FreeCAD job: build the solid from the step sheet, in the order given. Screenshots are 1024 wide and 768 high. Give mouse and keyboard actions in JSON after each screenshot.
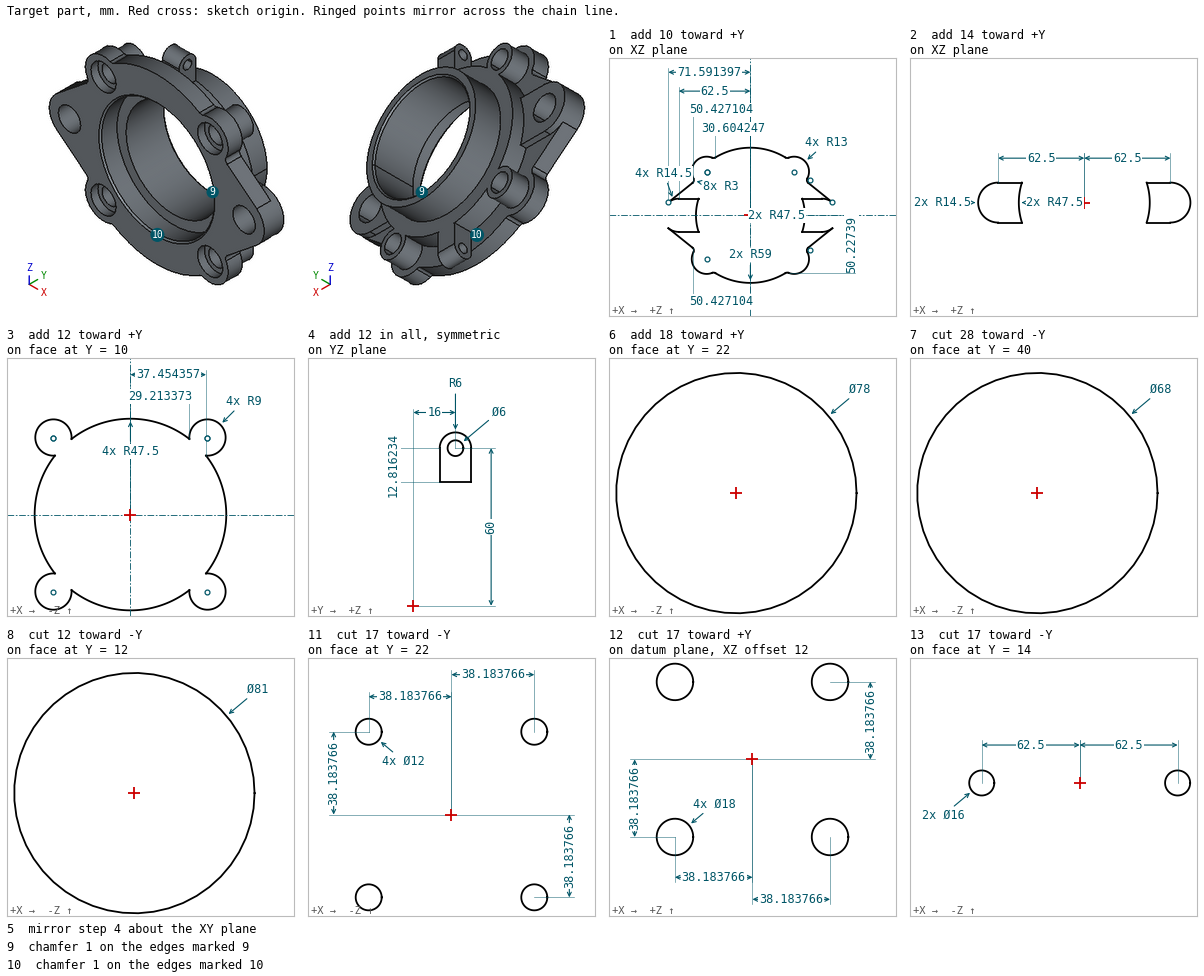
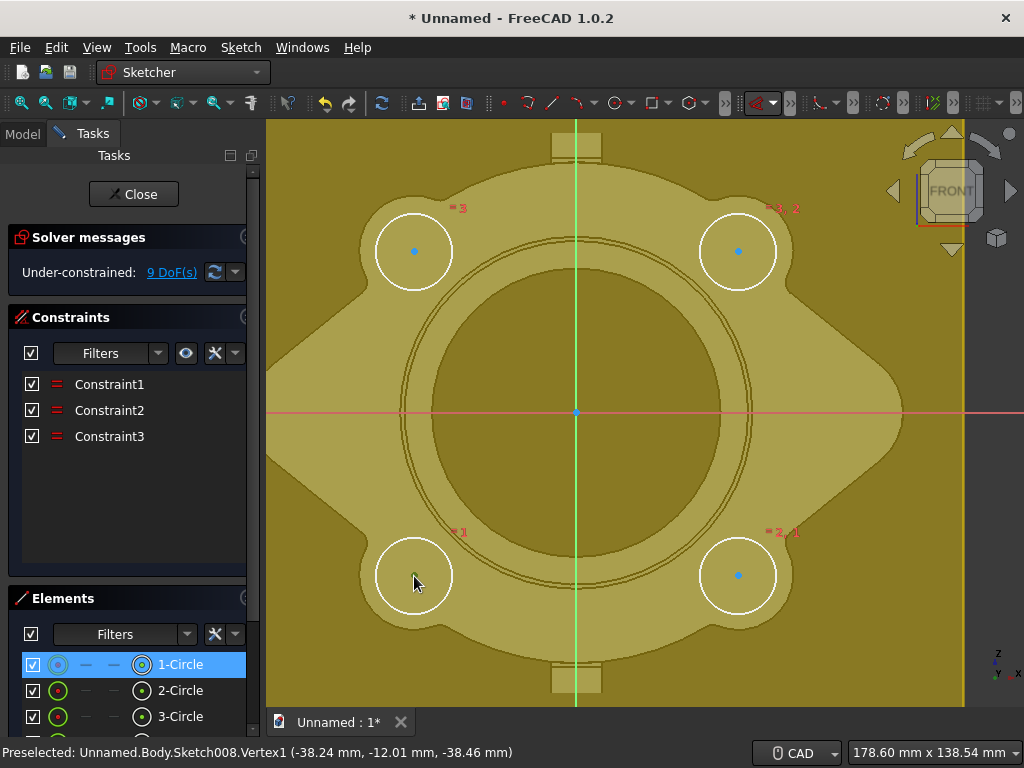
{"action": "left_click", "coordinate": [738, 576]}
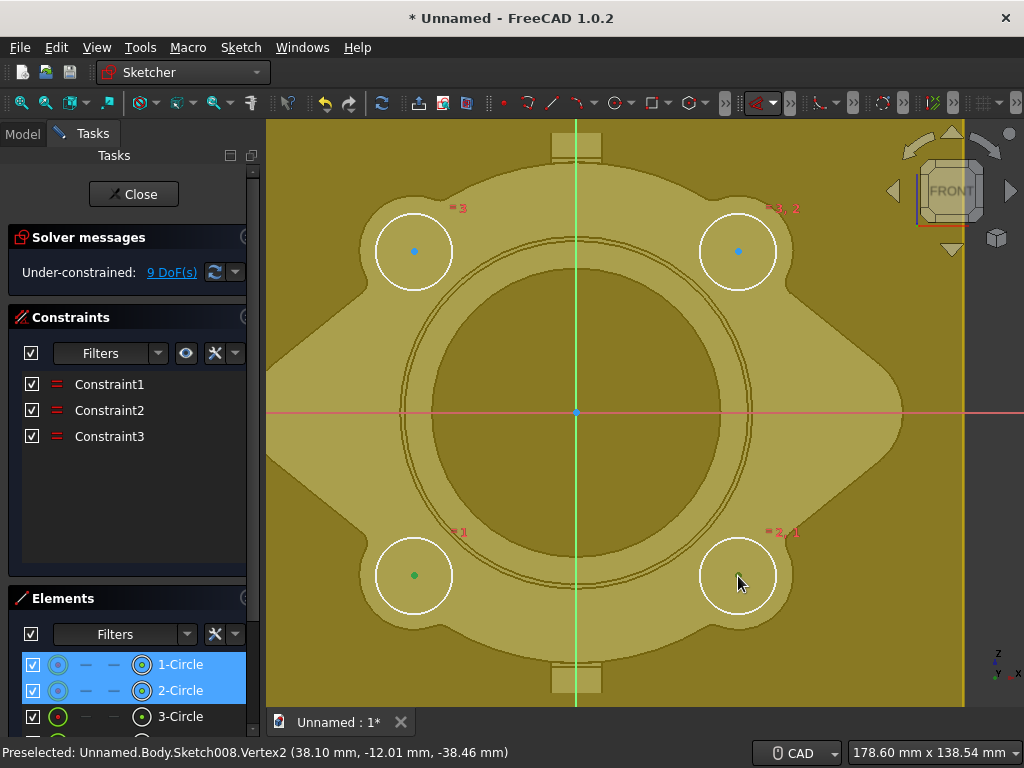
{"action": "key", "text": "h"}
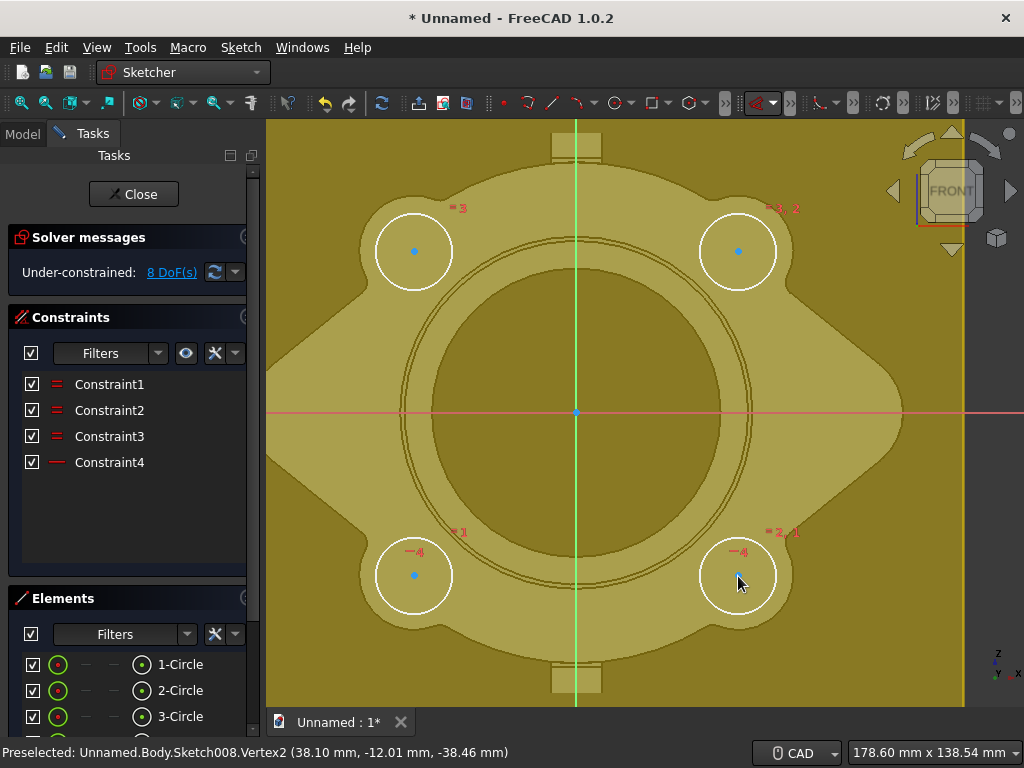
{"action": "left_click", "coordinate": [738, 576]}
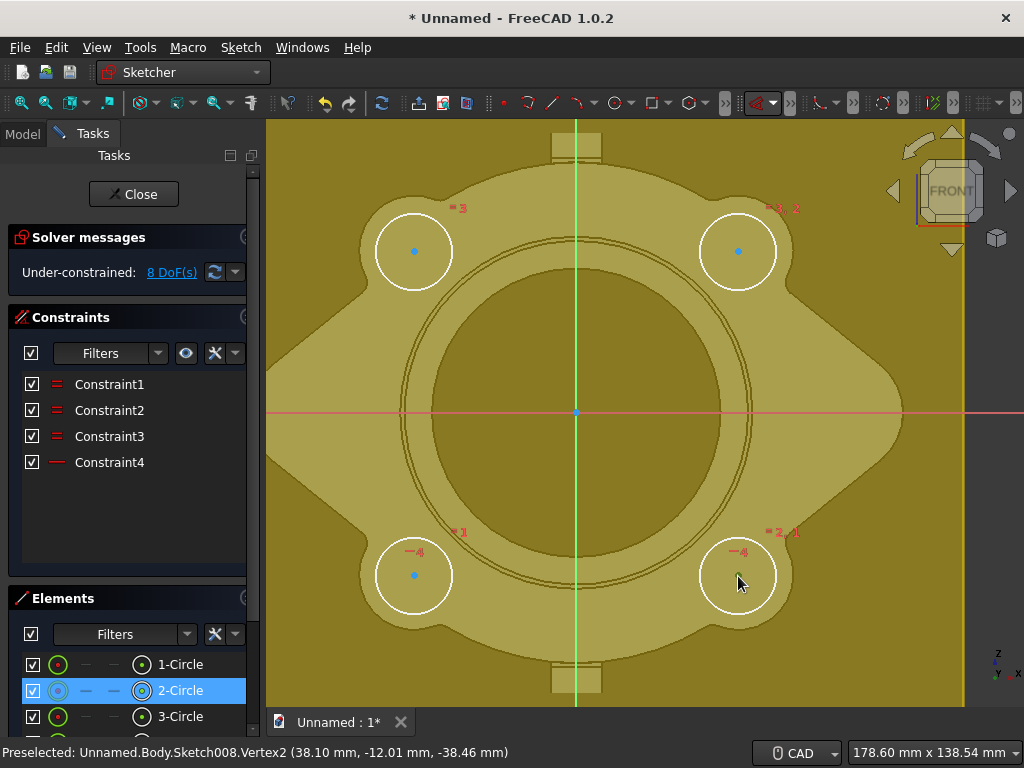
{"action": "left_click", "coordinate": [738, 252]}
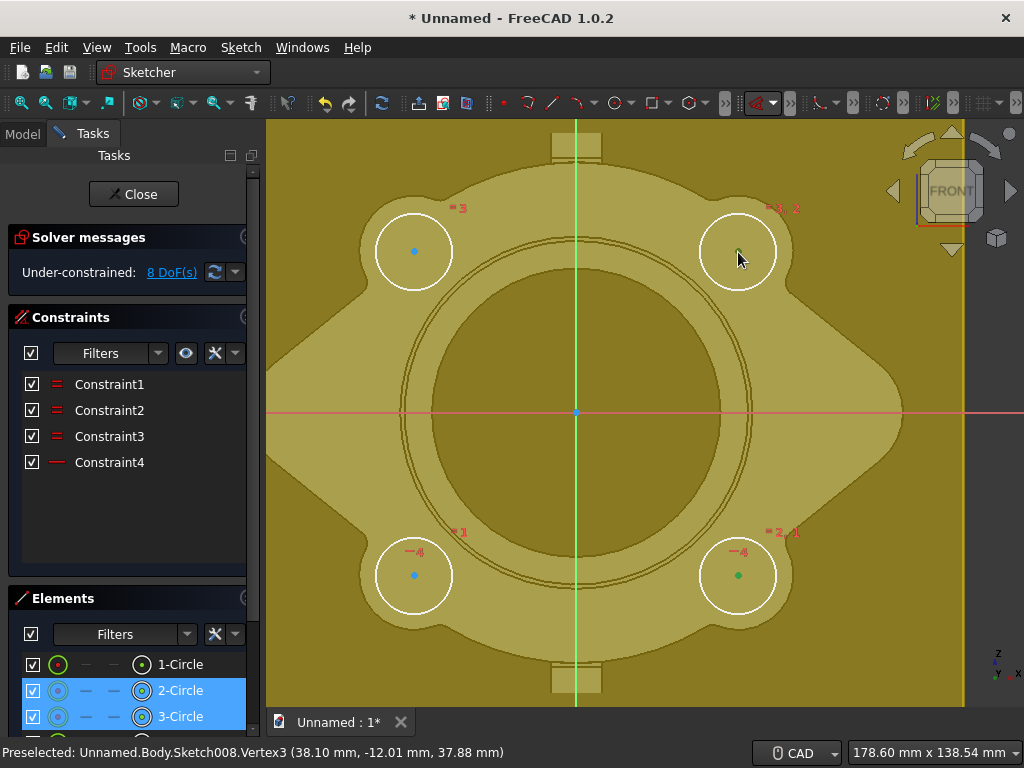
{"action": "key", "text": "v"}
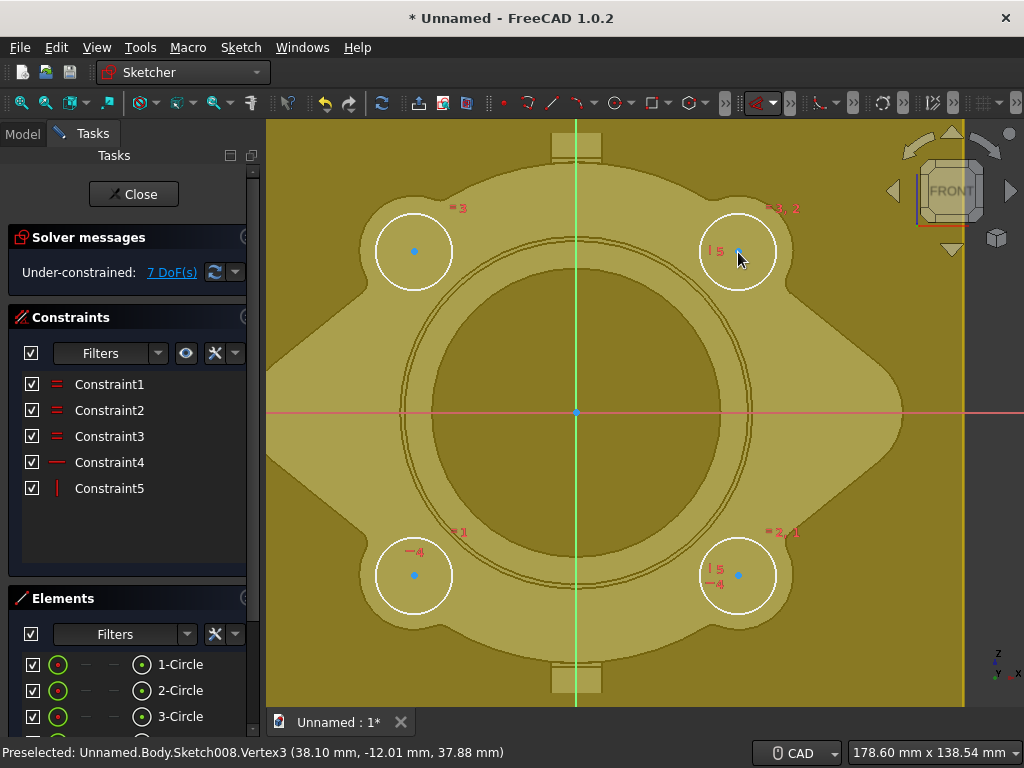
{"action": "left_click", "coordinate": [414, 576]}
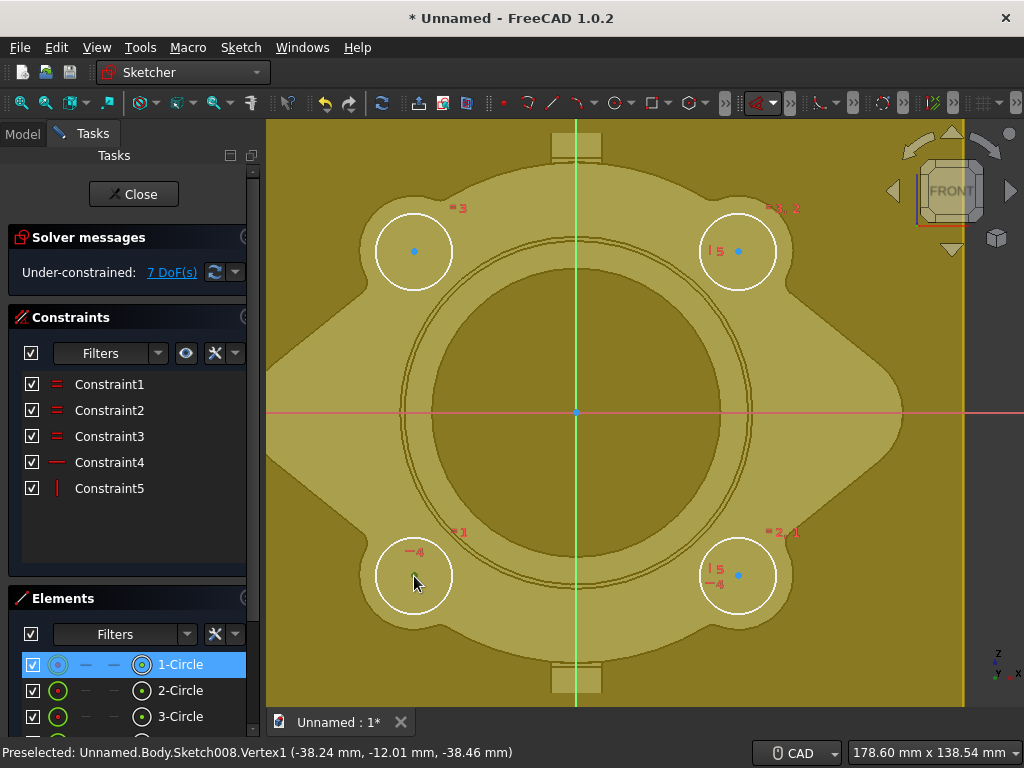
{"action": "left_click", "coordinate": [414, 252]}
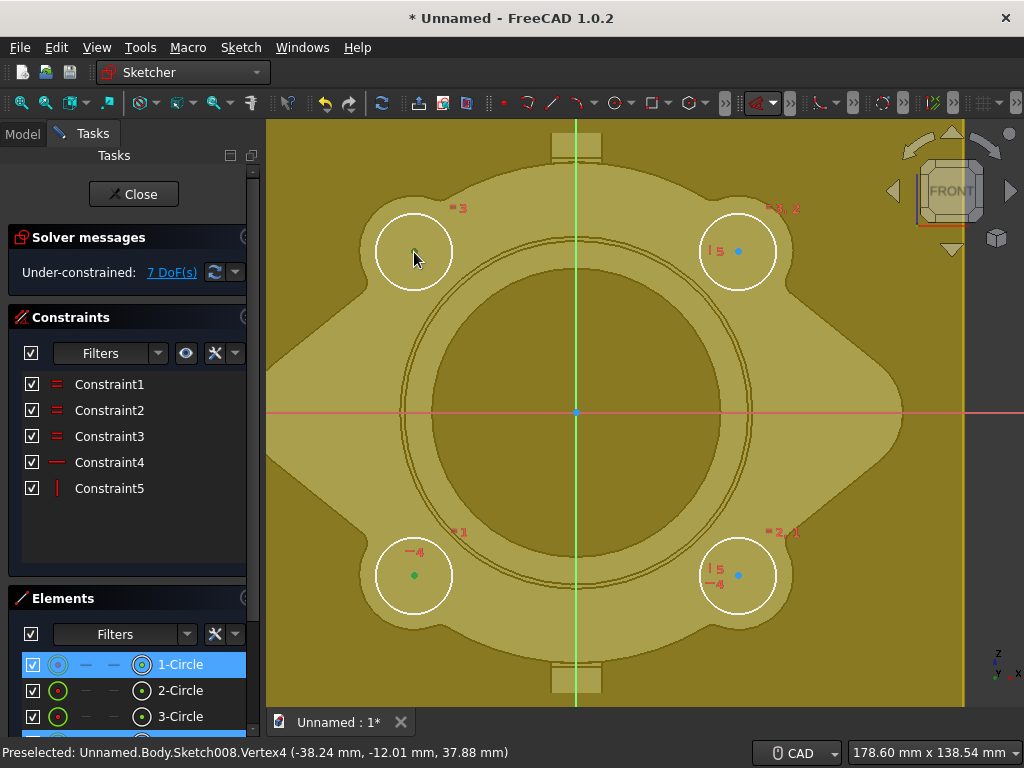
{"action": "key", "text": "v"}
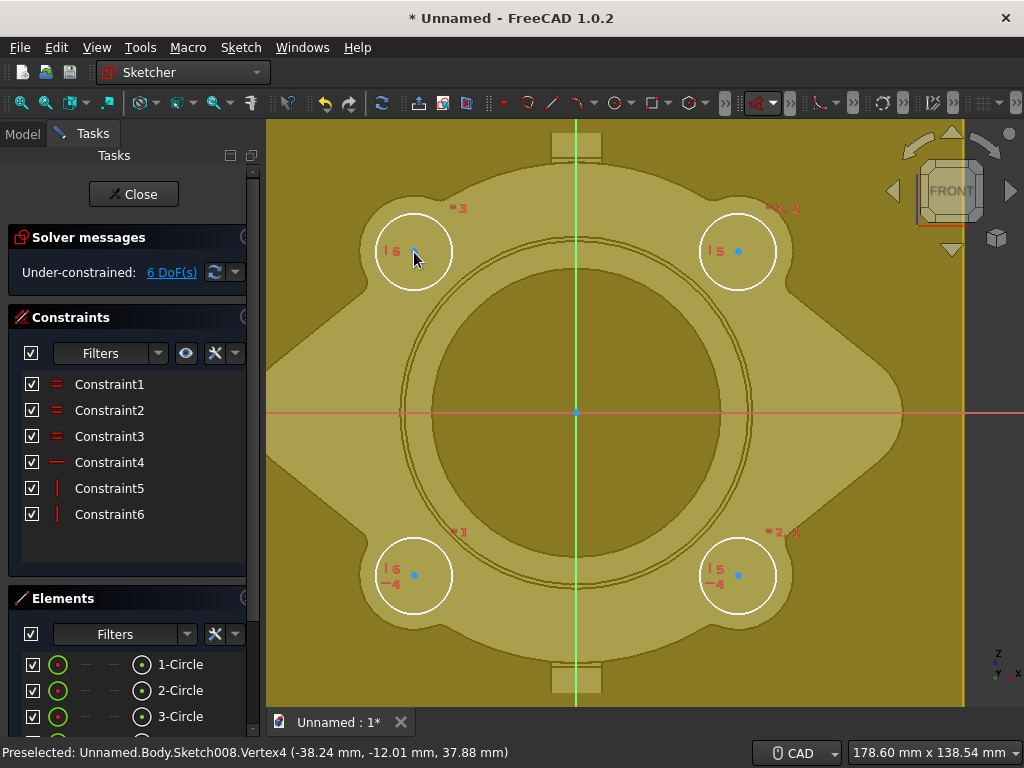
{"action": "left_click", "coordinate": [738, 252]}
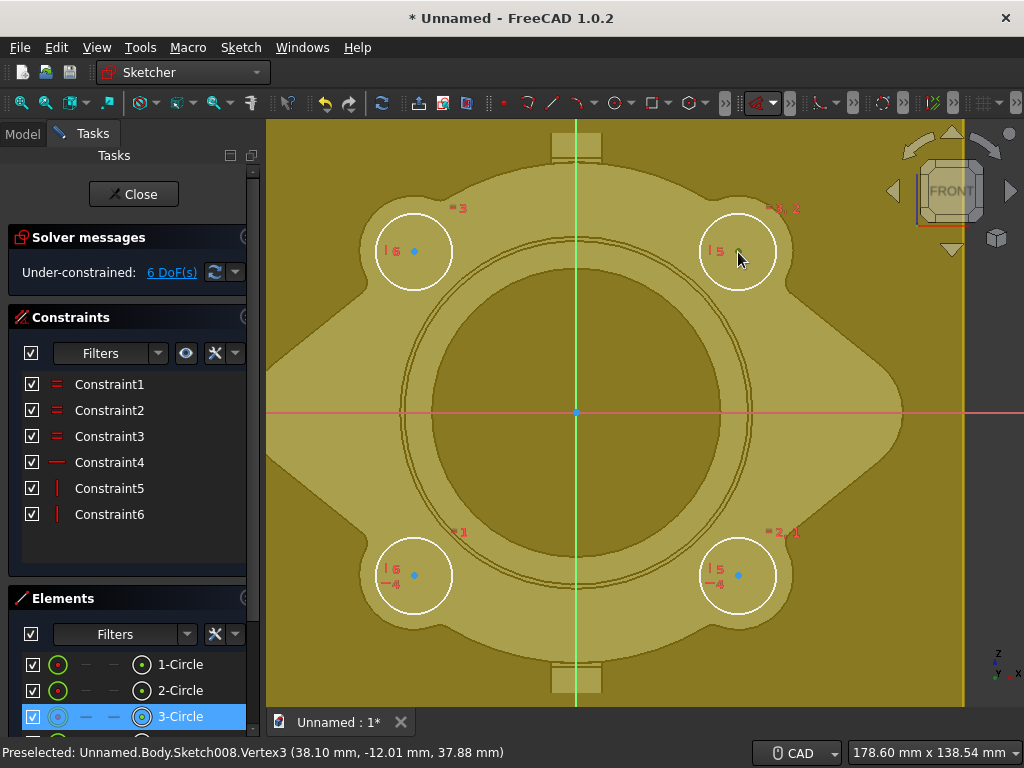
{"action": "left_click", "coordinate": [414, 252]}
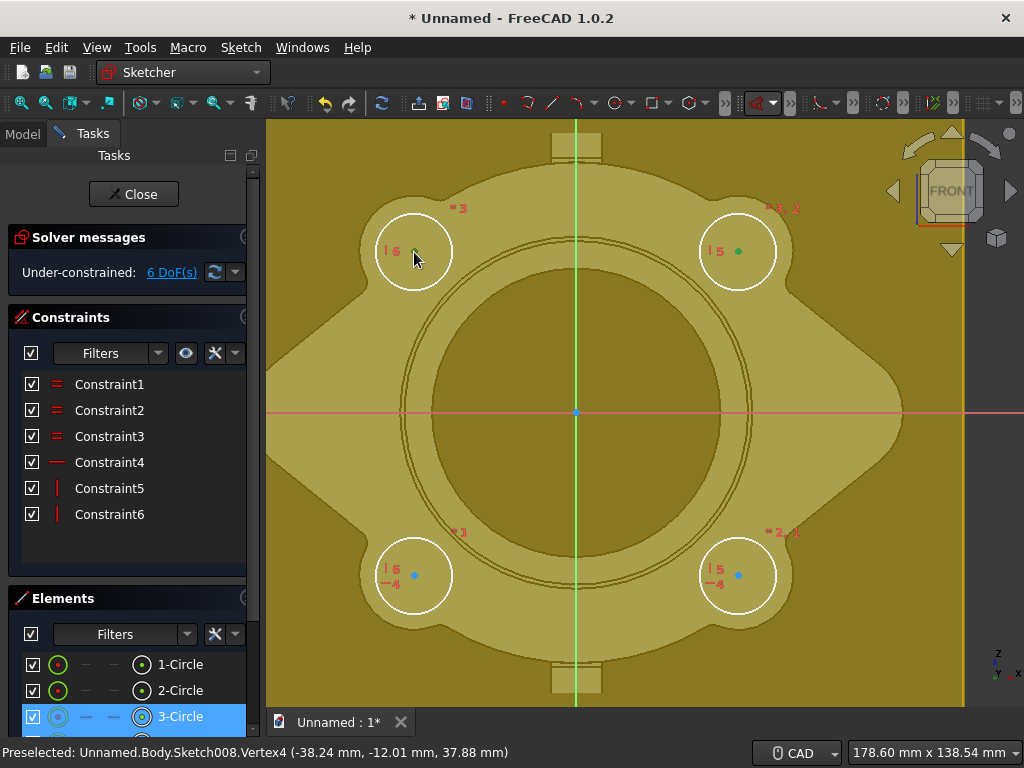
{"action": "key", "text": "h"}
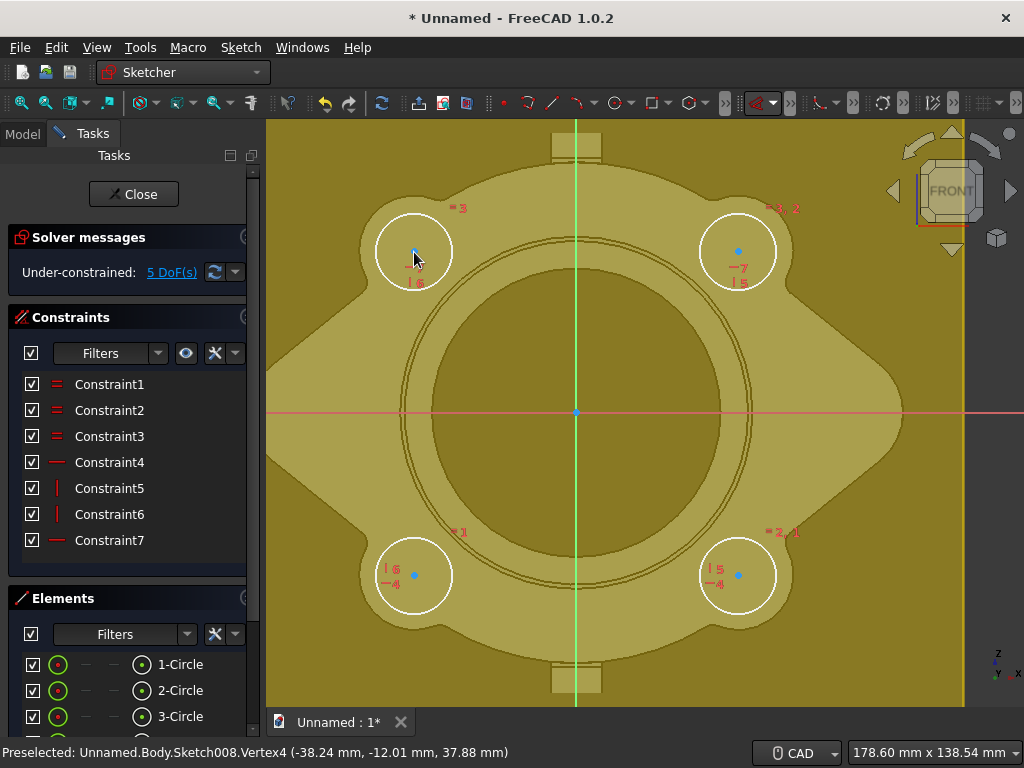
{"action": "key", "text": "d"}